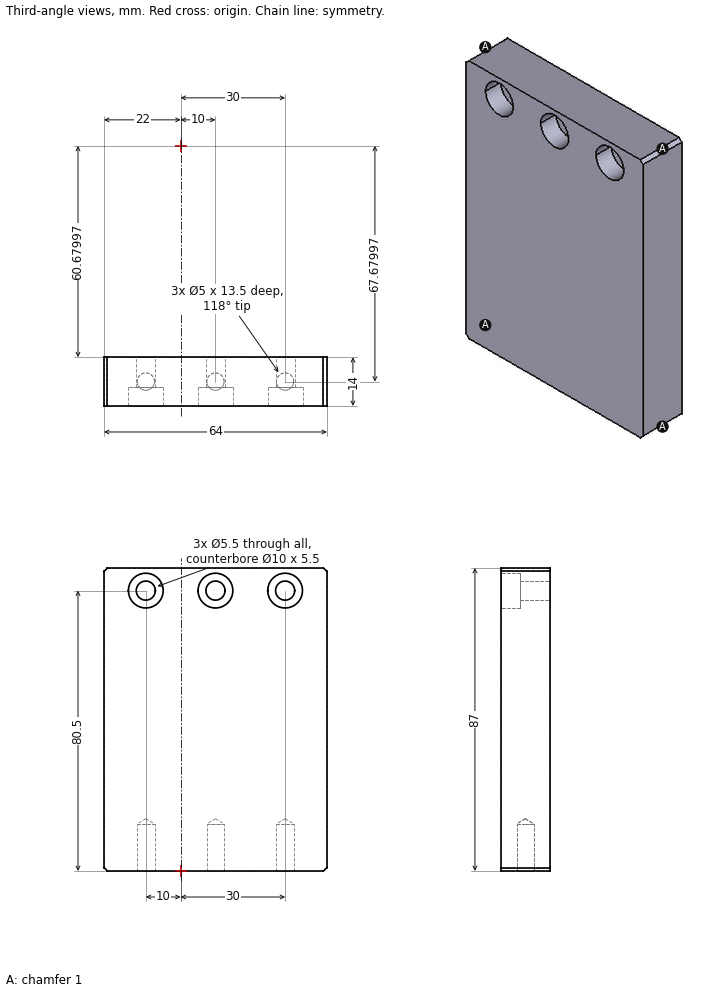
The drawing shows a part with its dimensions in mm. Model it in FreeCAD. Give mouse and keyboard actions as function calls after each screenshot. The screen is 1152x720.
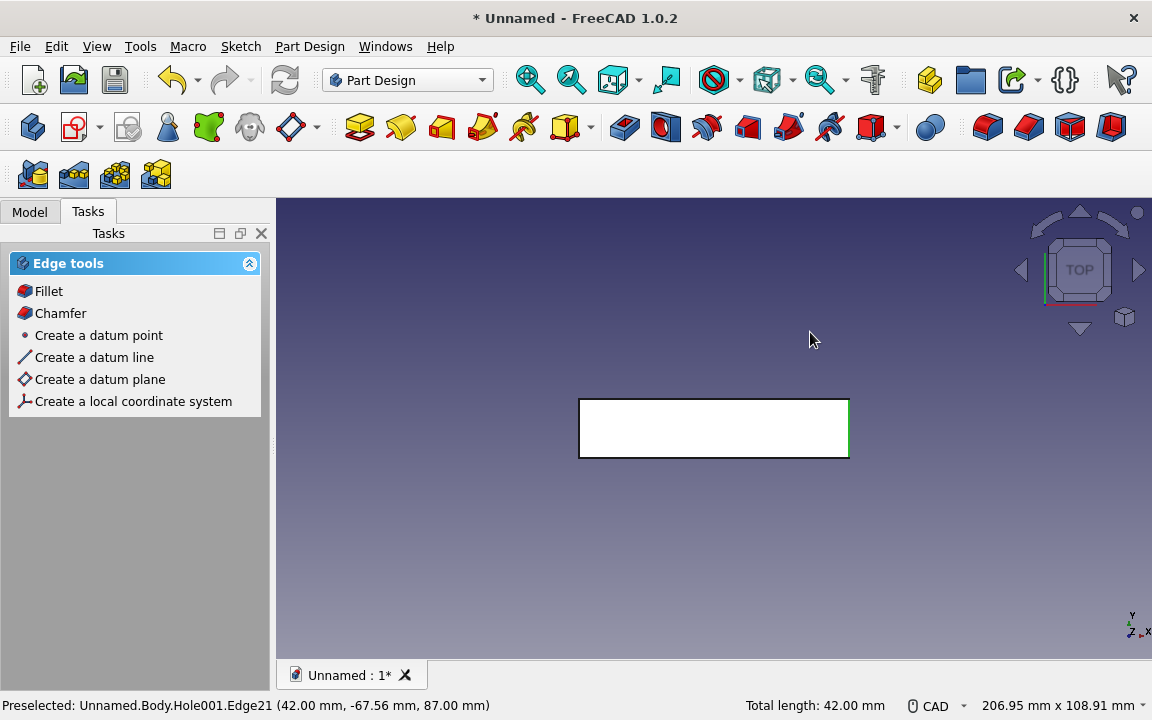
key(v)
key(f)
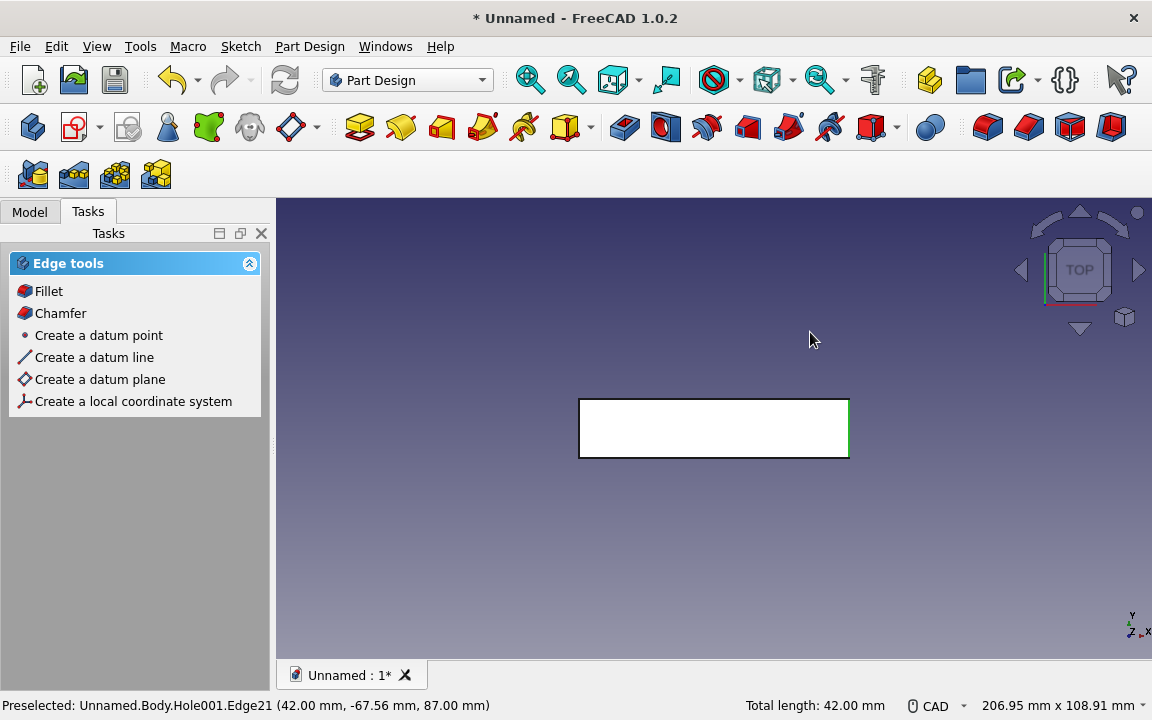
click(579, 427, ctrl)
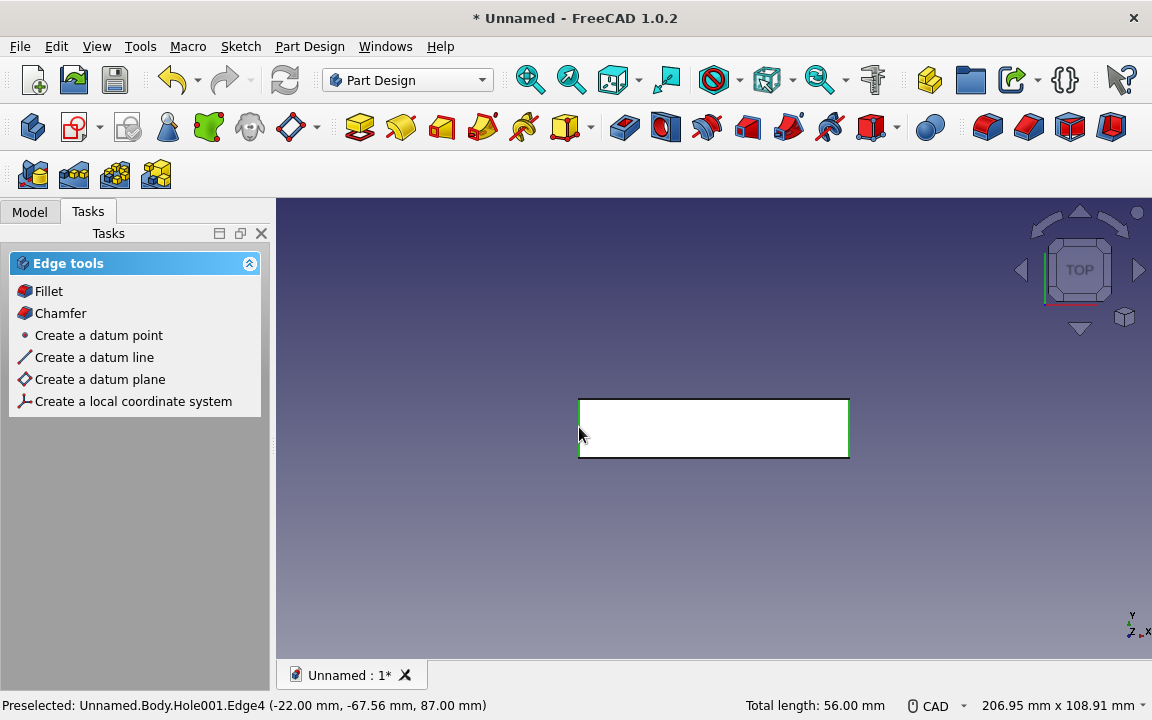
click(1029, 128)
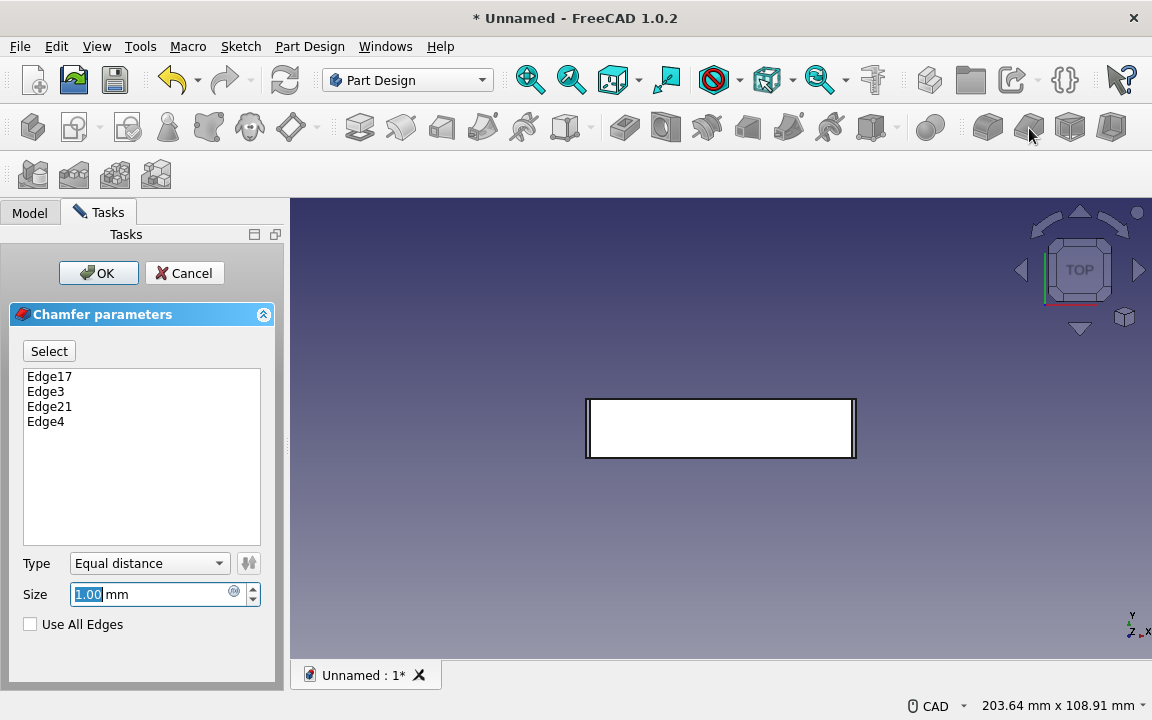
text(1)
key(Tab)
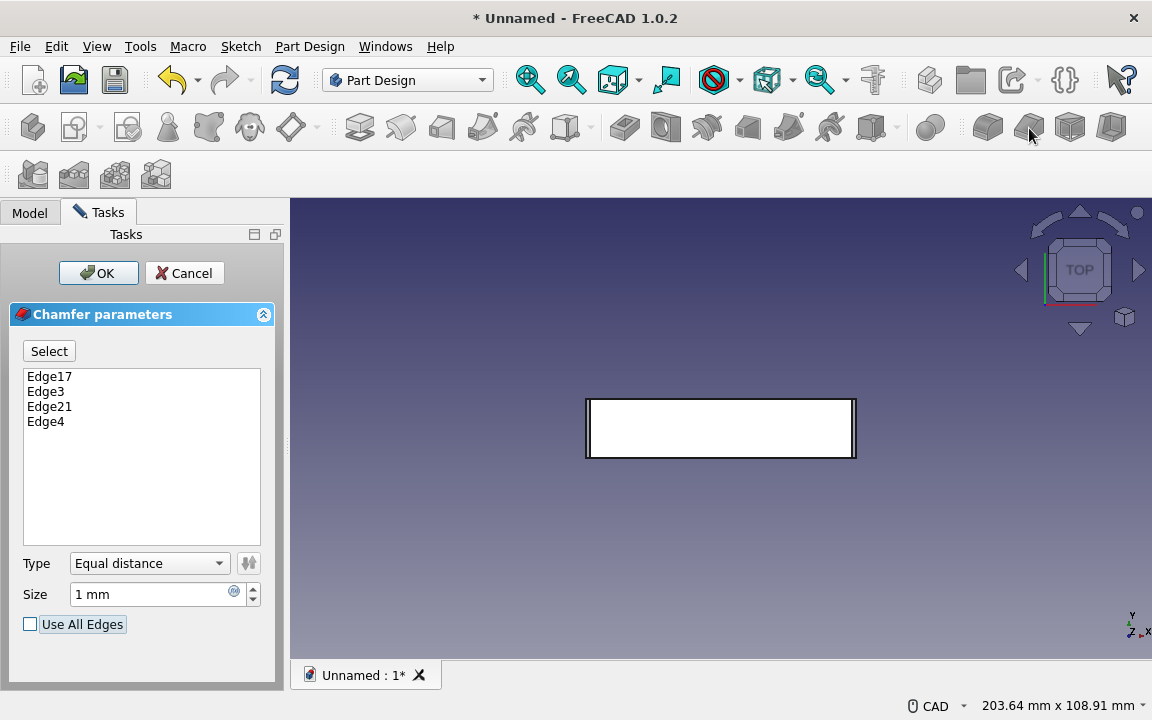
click(99, 273)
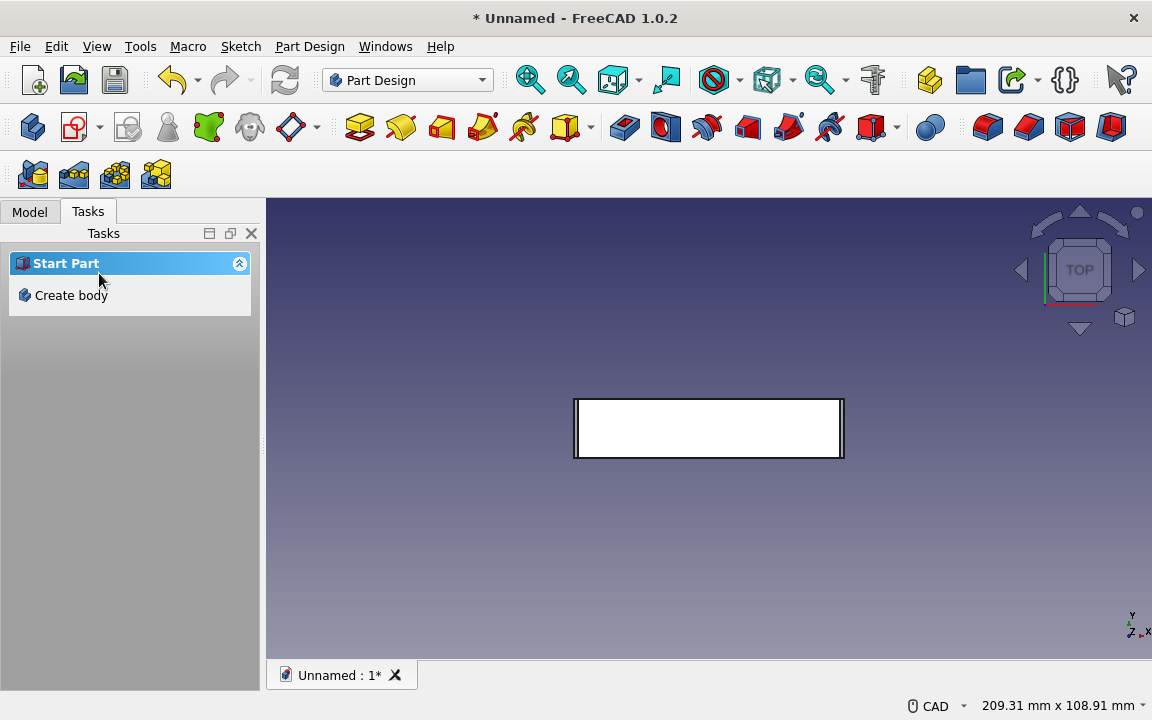
key(0)